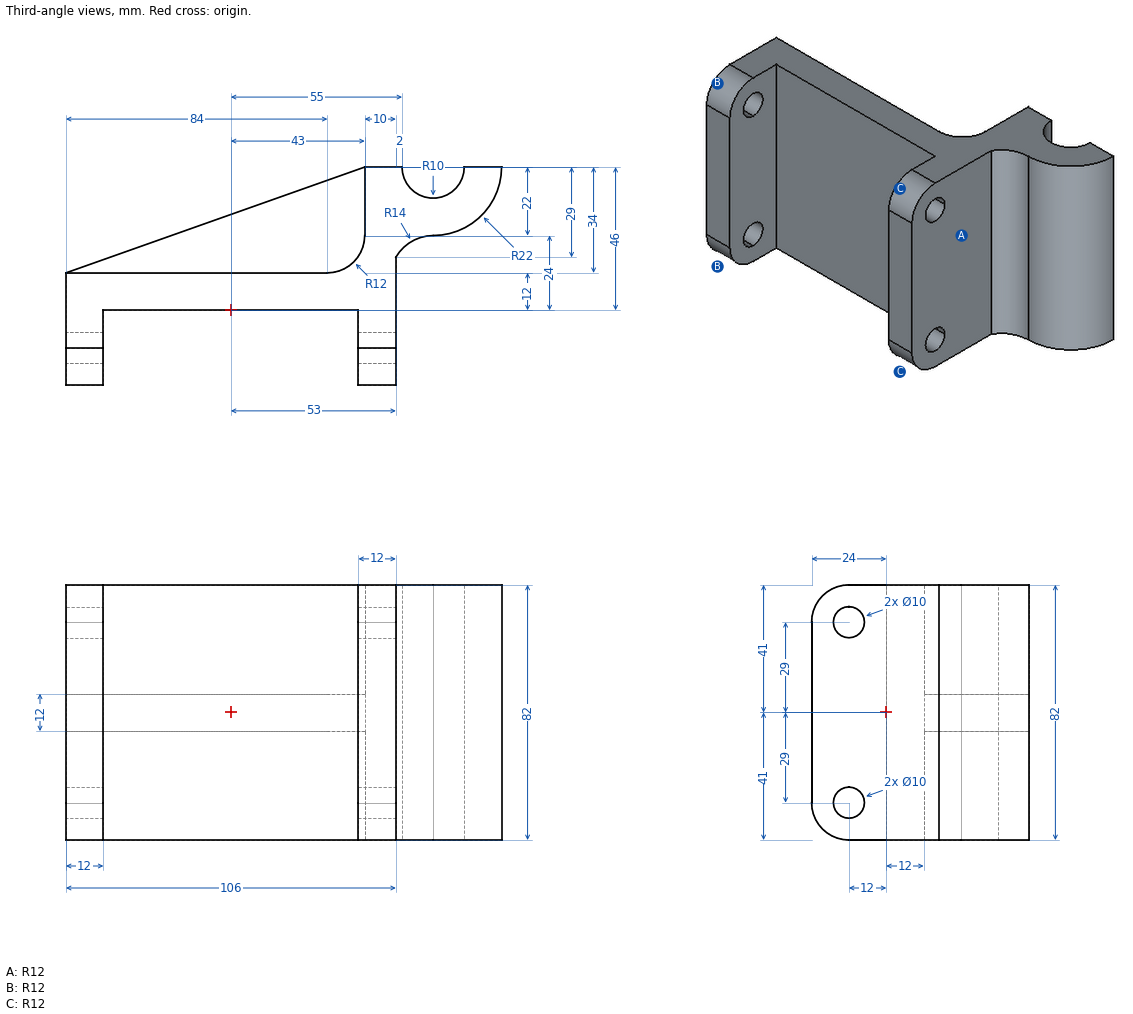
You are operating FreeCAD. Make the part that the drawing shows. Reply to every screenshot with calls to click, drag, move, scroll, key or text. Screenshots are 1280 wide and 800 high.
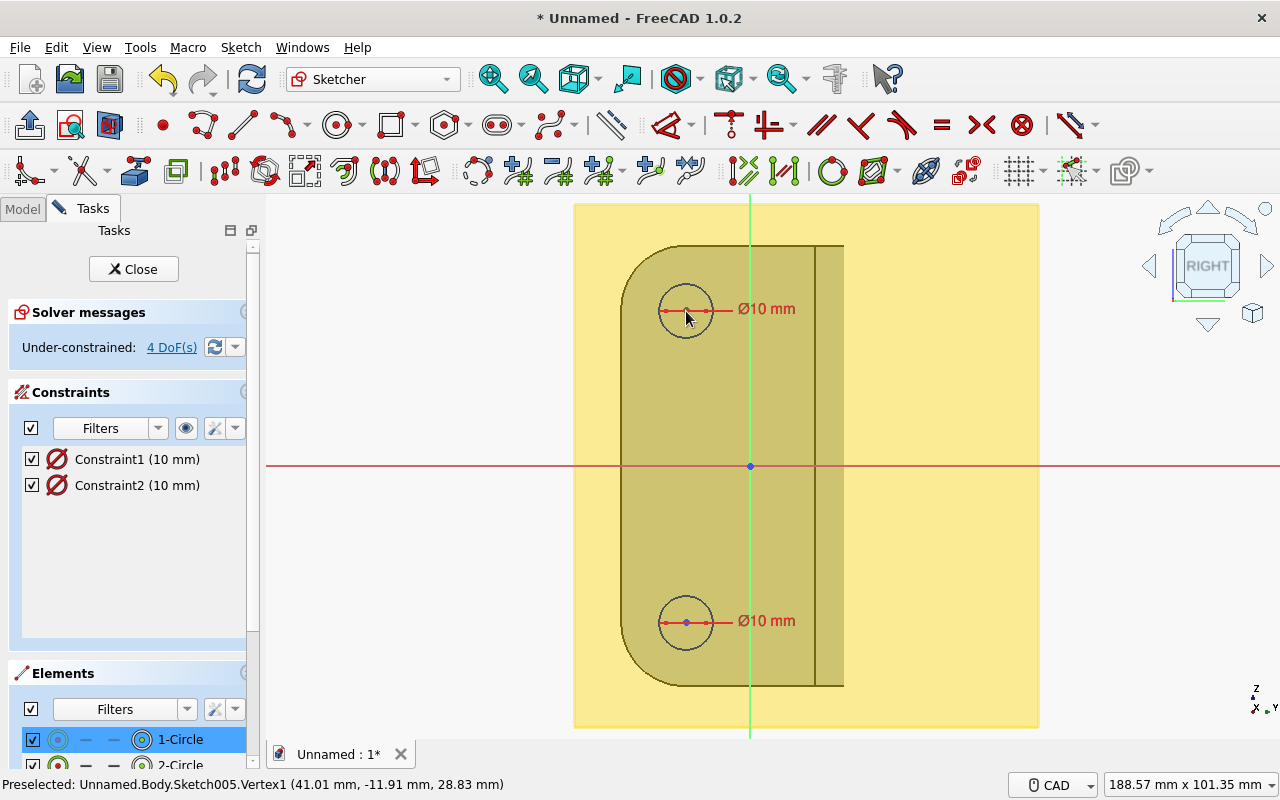
click(686, 623)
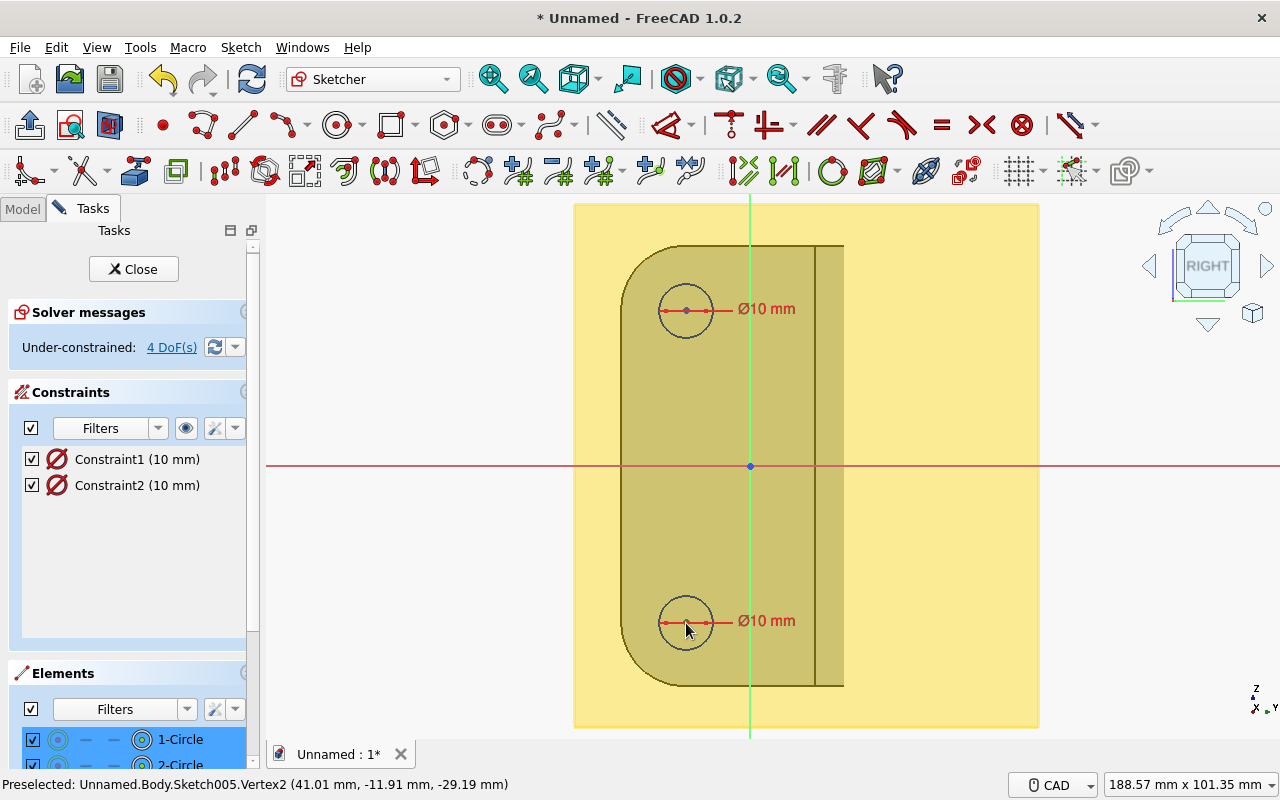
click(796, 126)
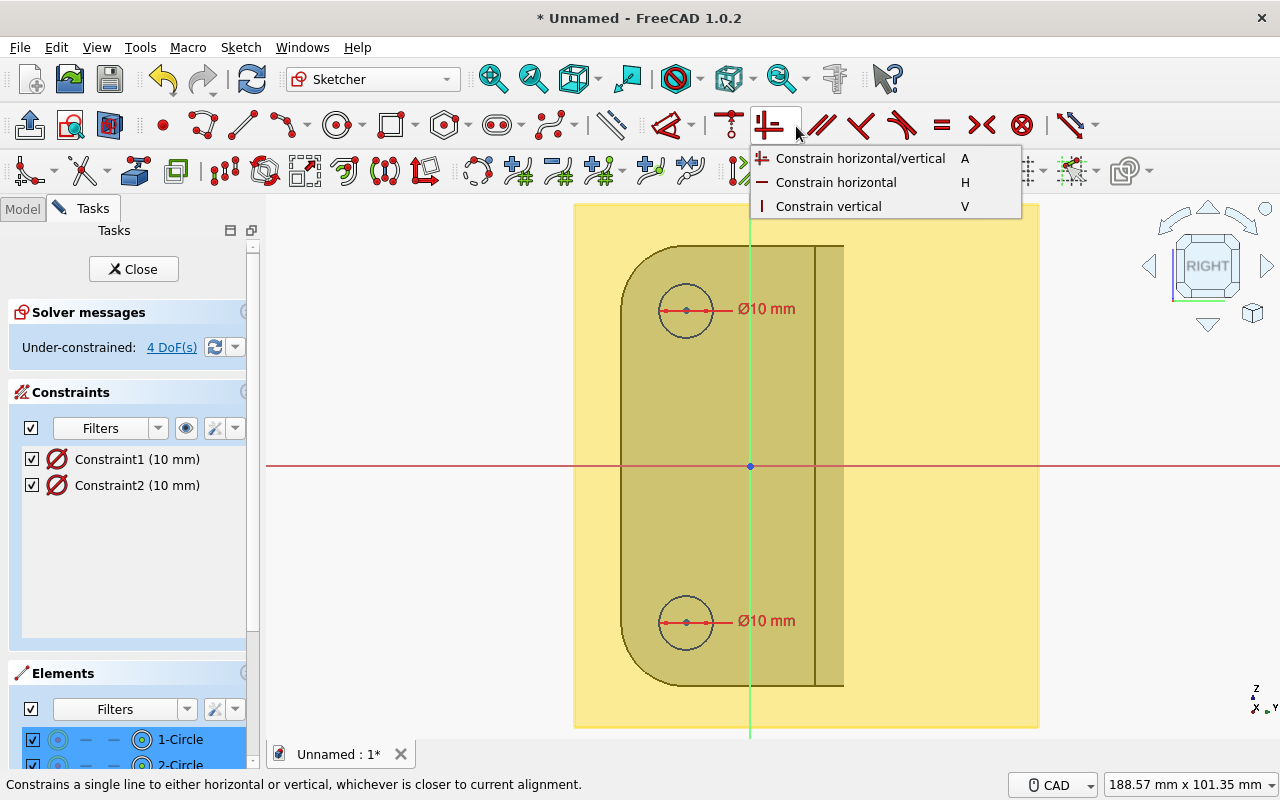
click(886, 206)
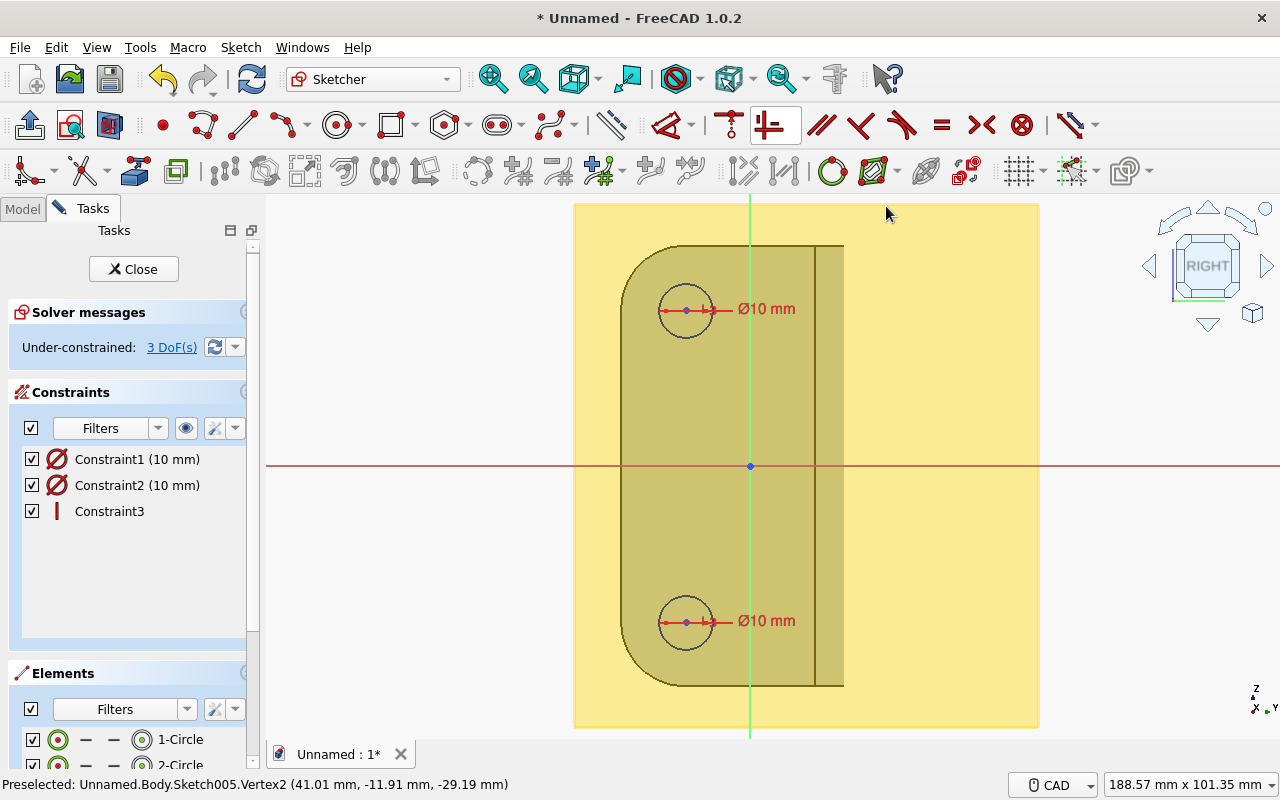
key(d)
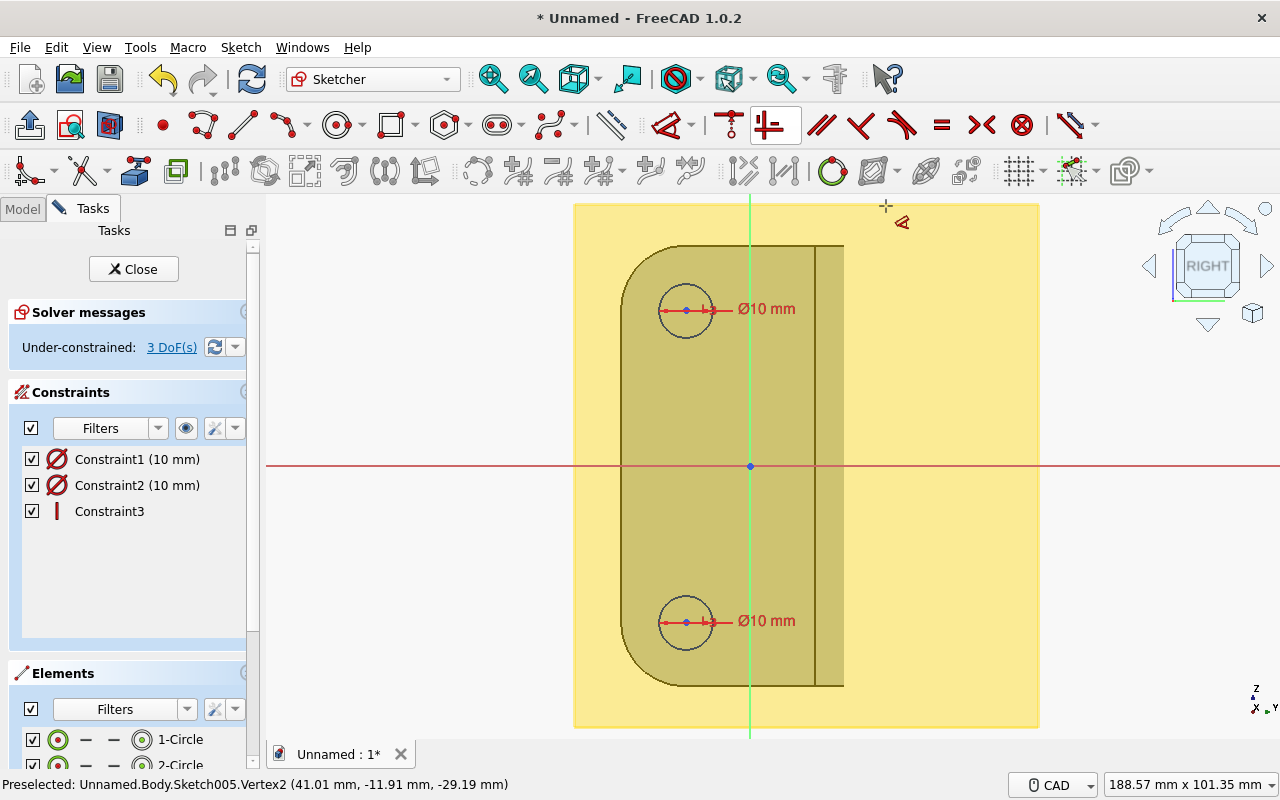
click(686, 311)
click(718, 277)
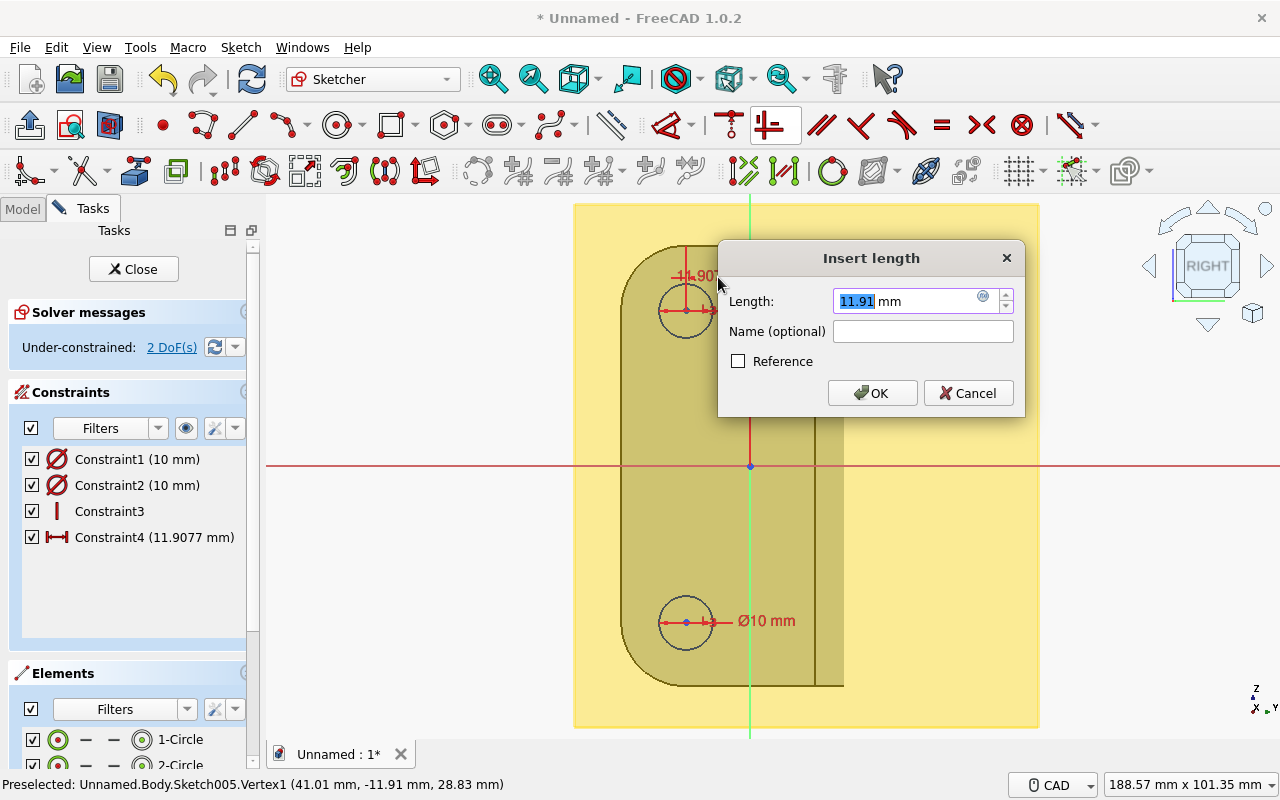
text(12)
key(Return)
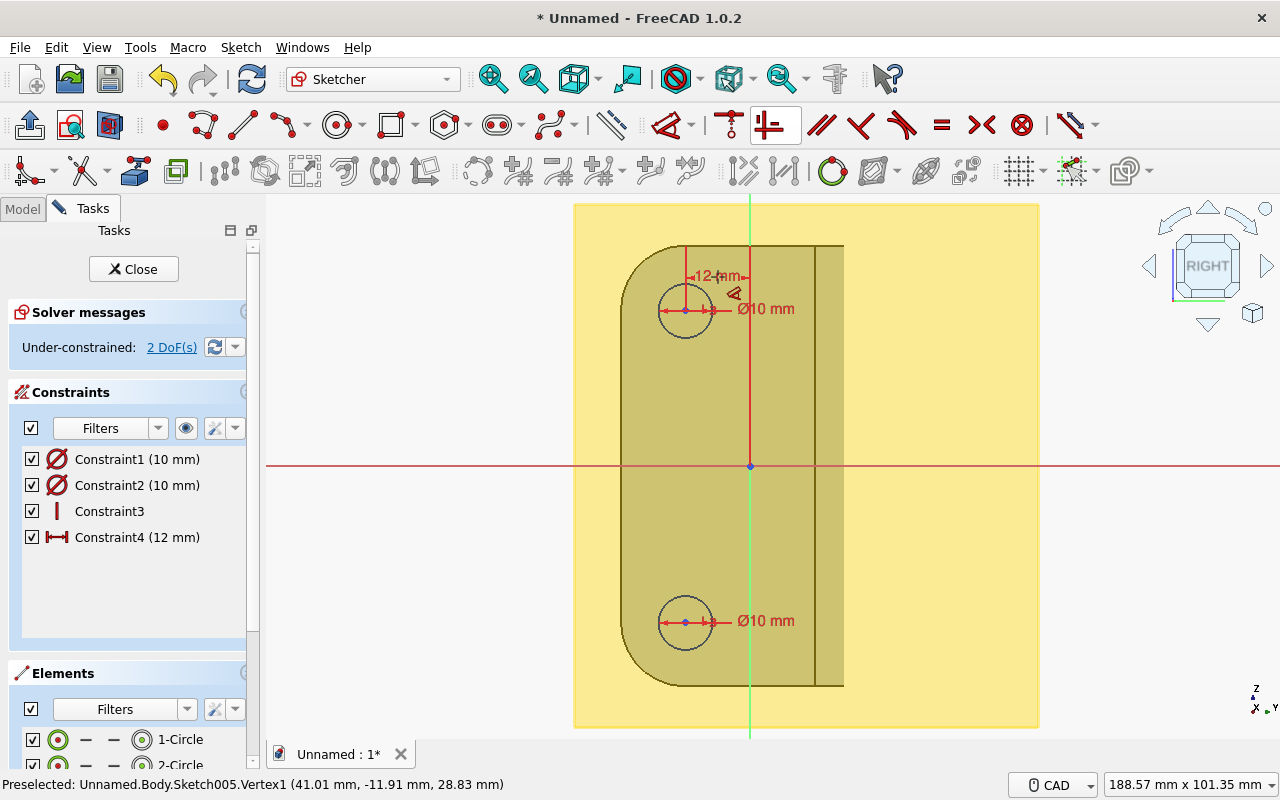
click(686, 311)
click(784, 389)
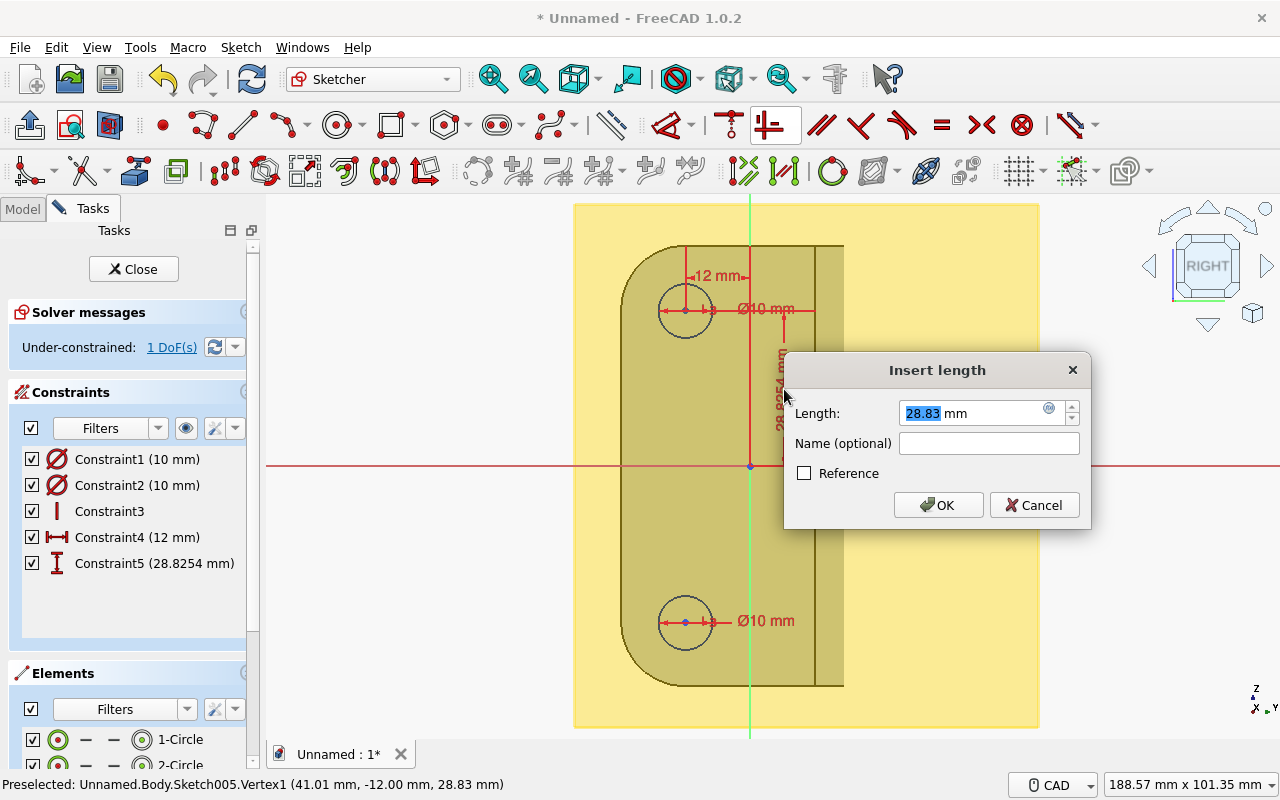
text(29)
key(Return)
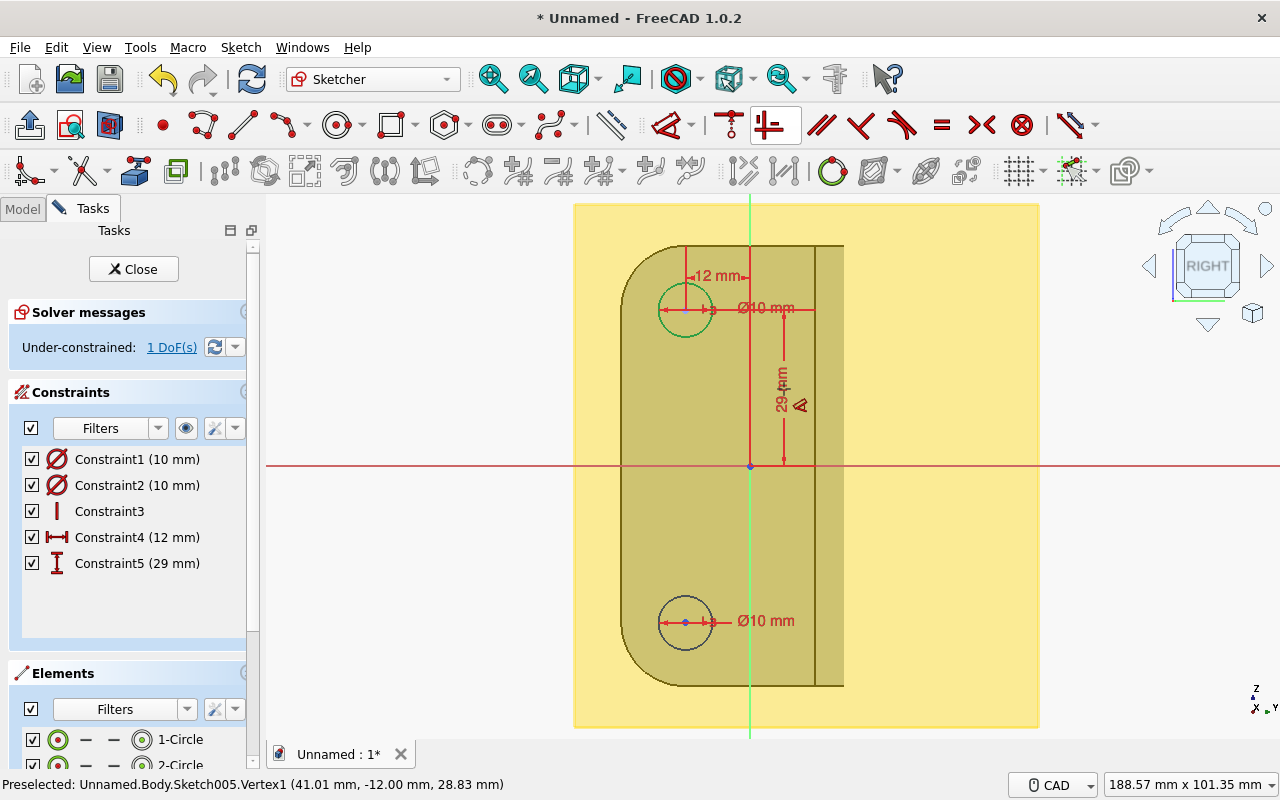
click(686, 623)
click(784, 545)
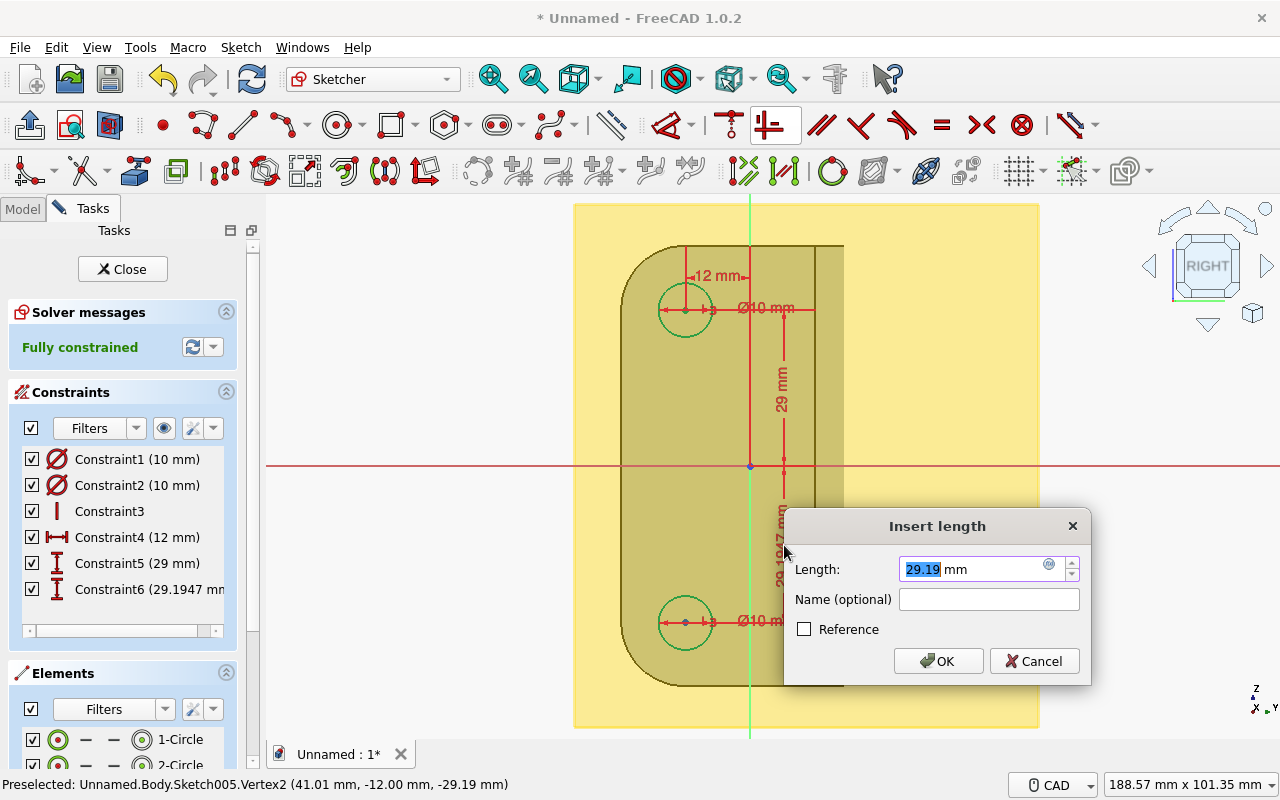
text(29)
key(Return)
key(Escape)